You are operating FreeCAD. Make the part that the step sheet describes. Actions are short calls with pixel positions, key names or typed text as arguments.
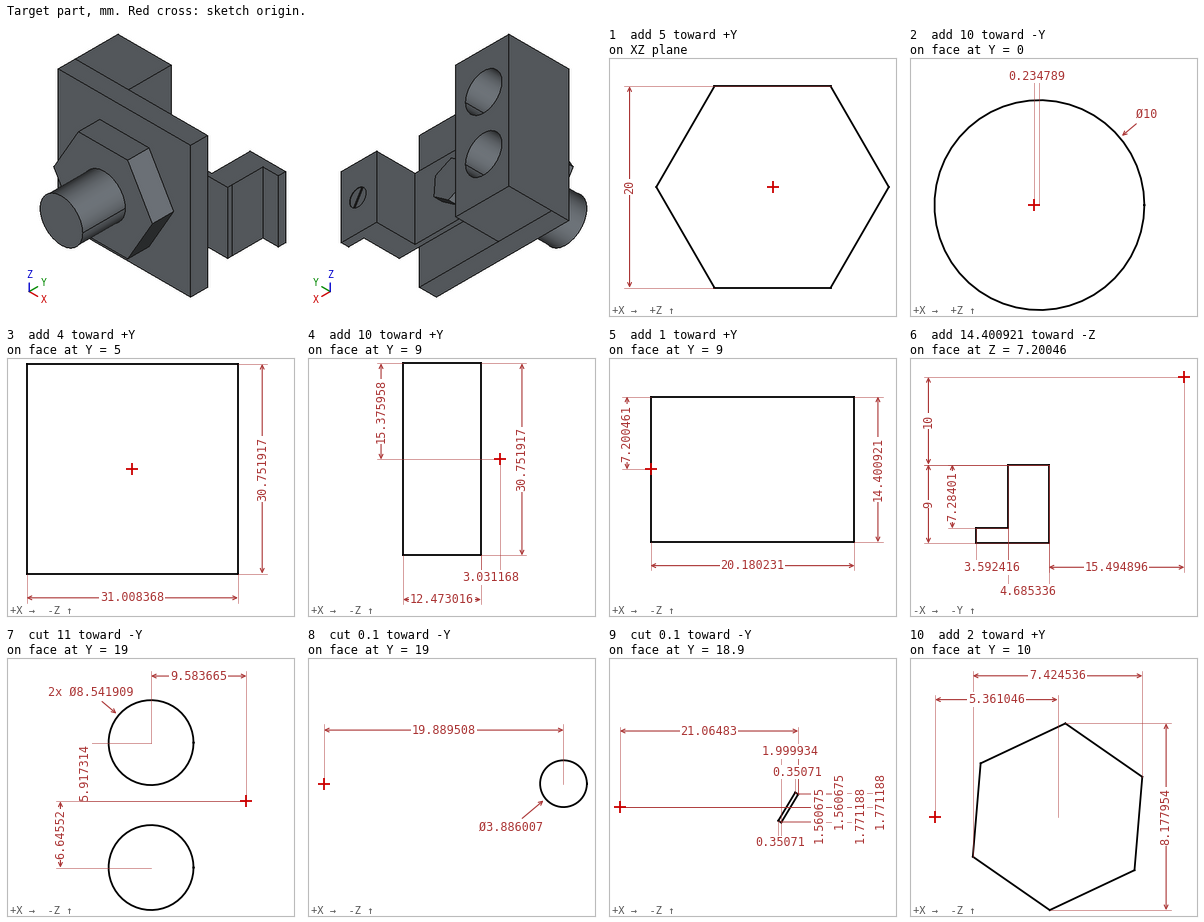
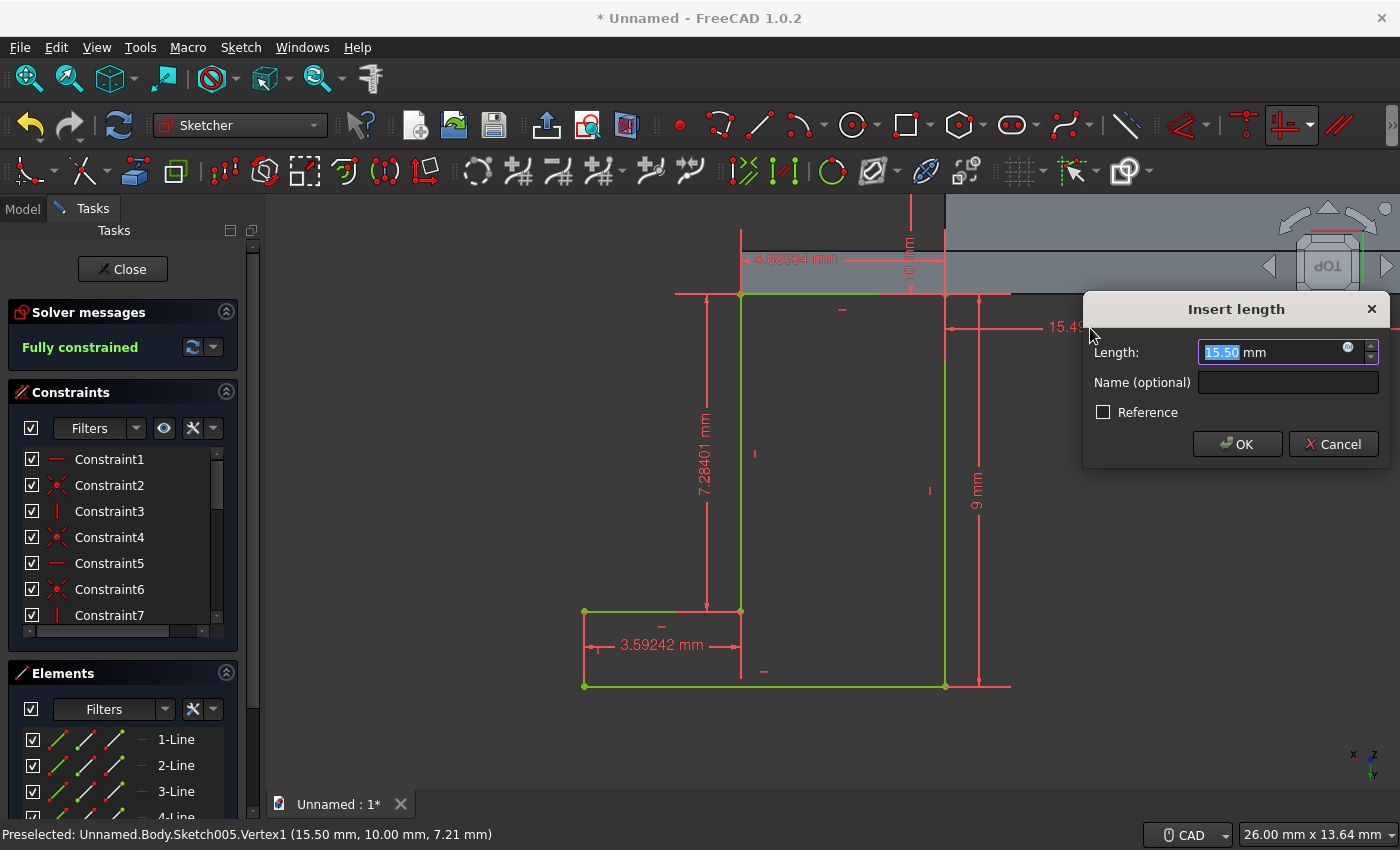
text(15.494896)
key(Return)
key(Escape)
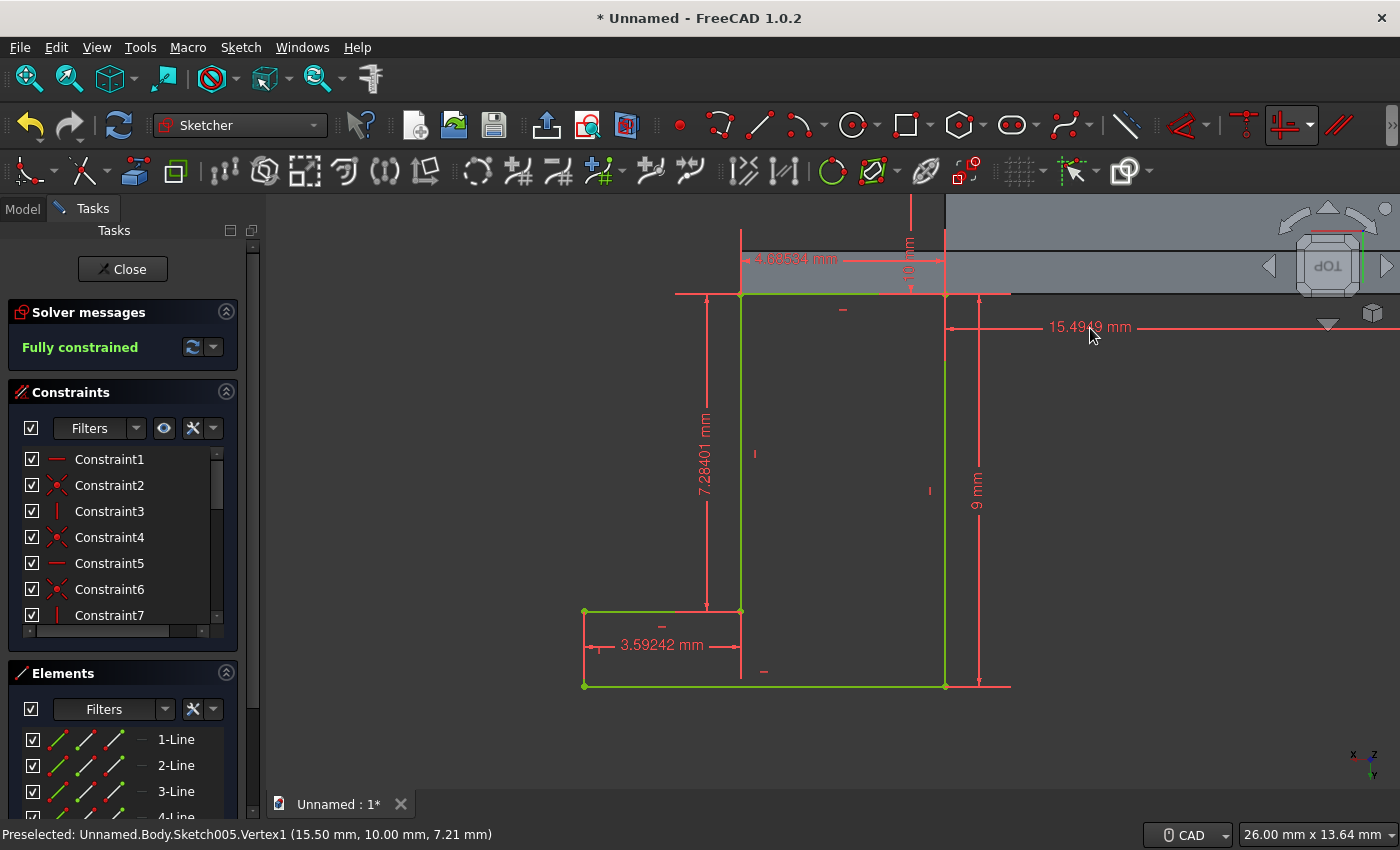
click(123, 269)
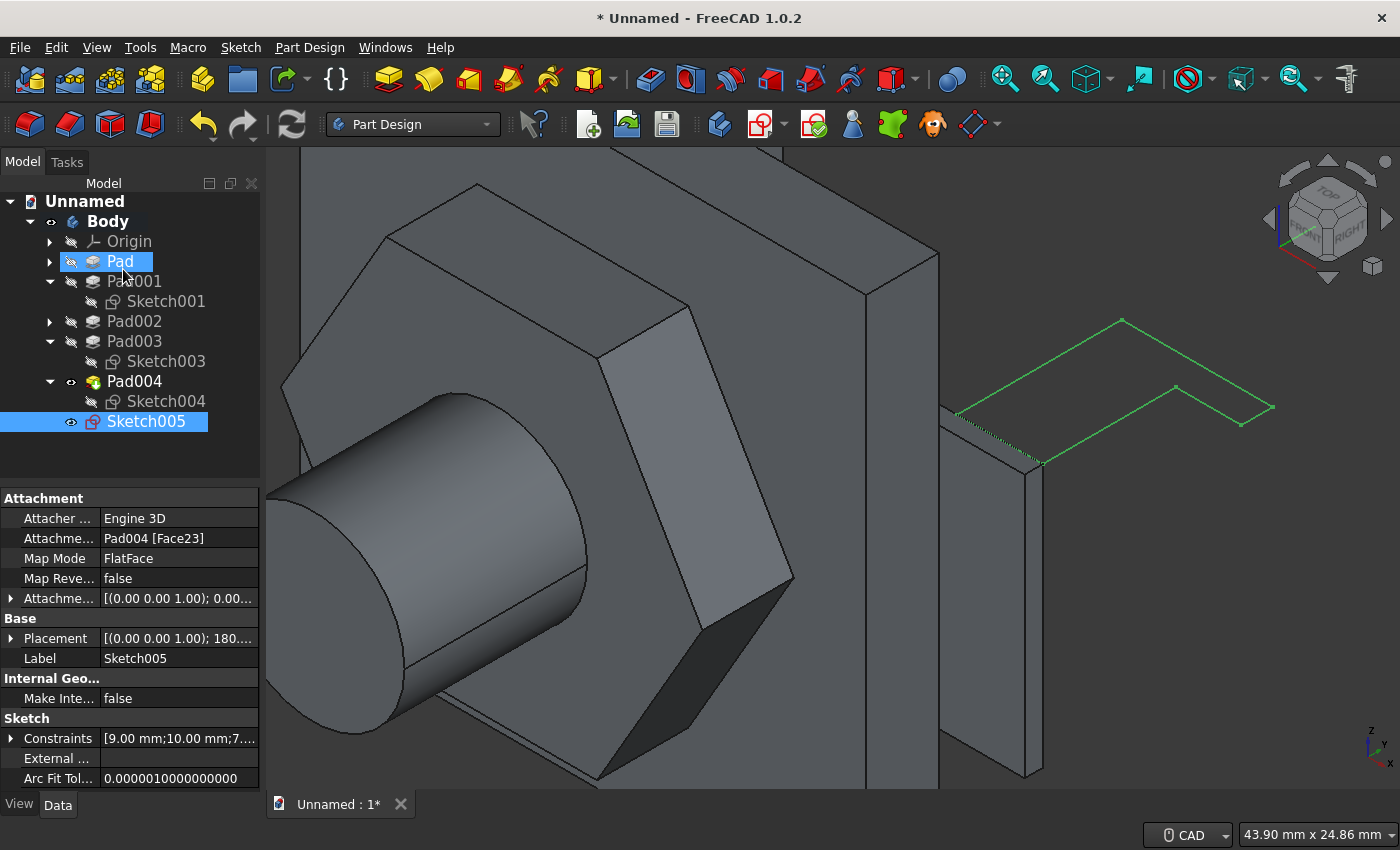
click(390, 80)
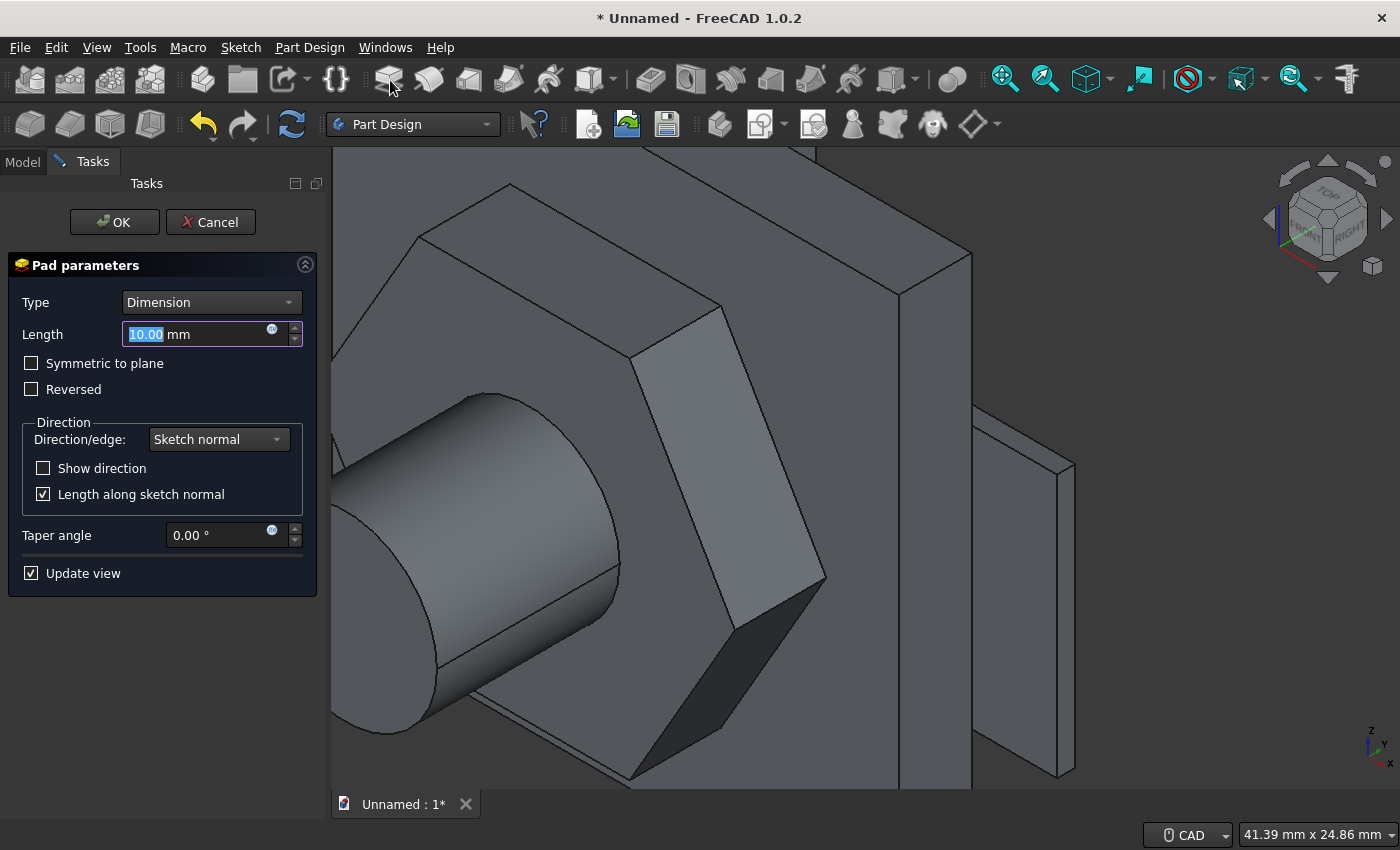
text(14.400921)
key(Tab)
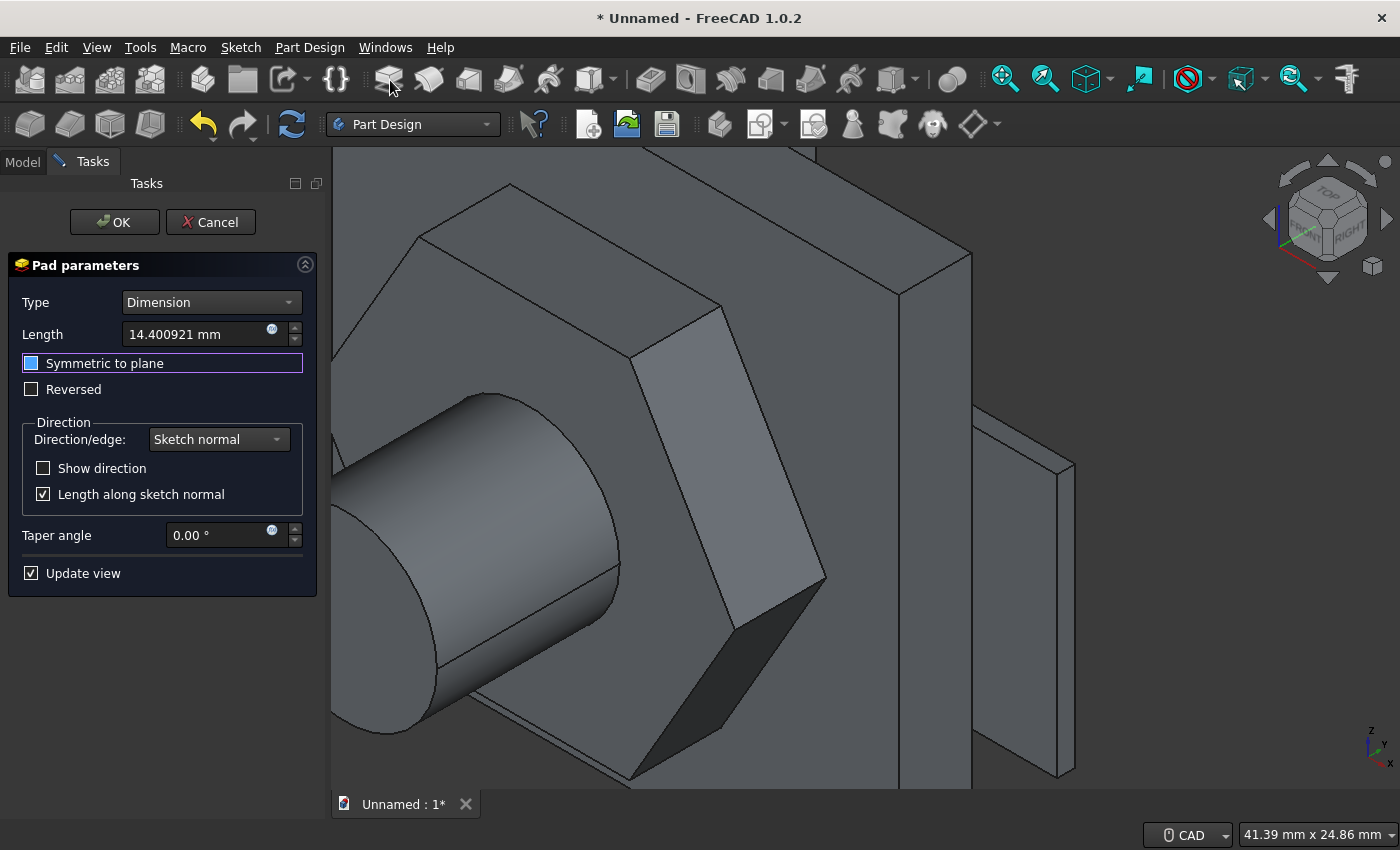
click(30, 389)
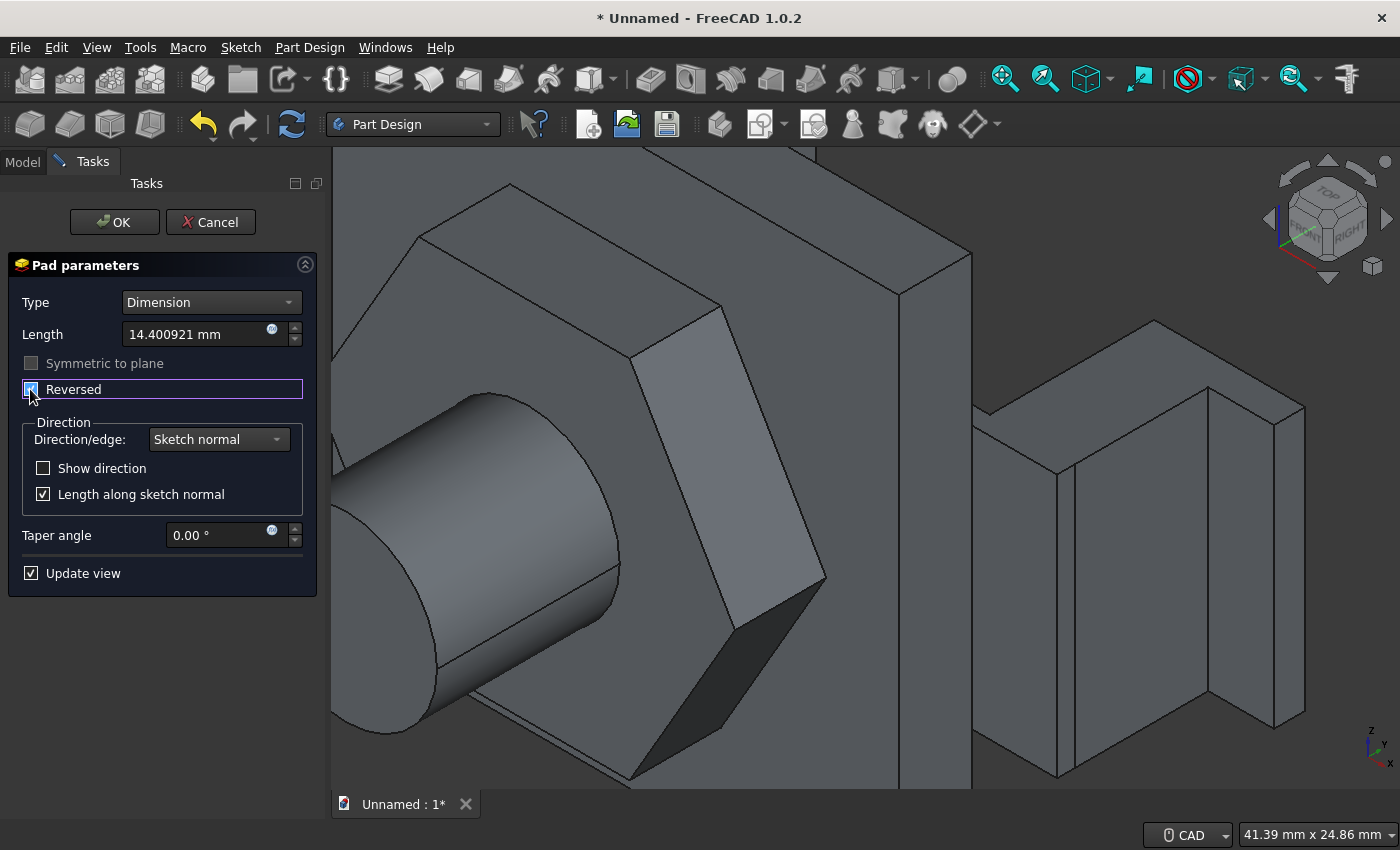
click(115, 222)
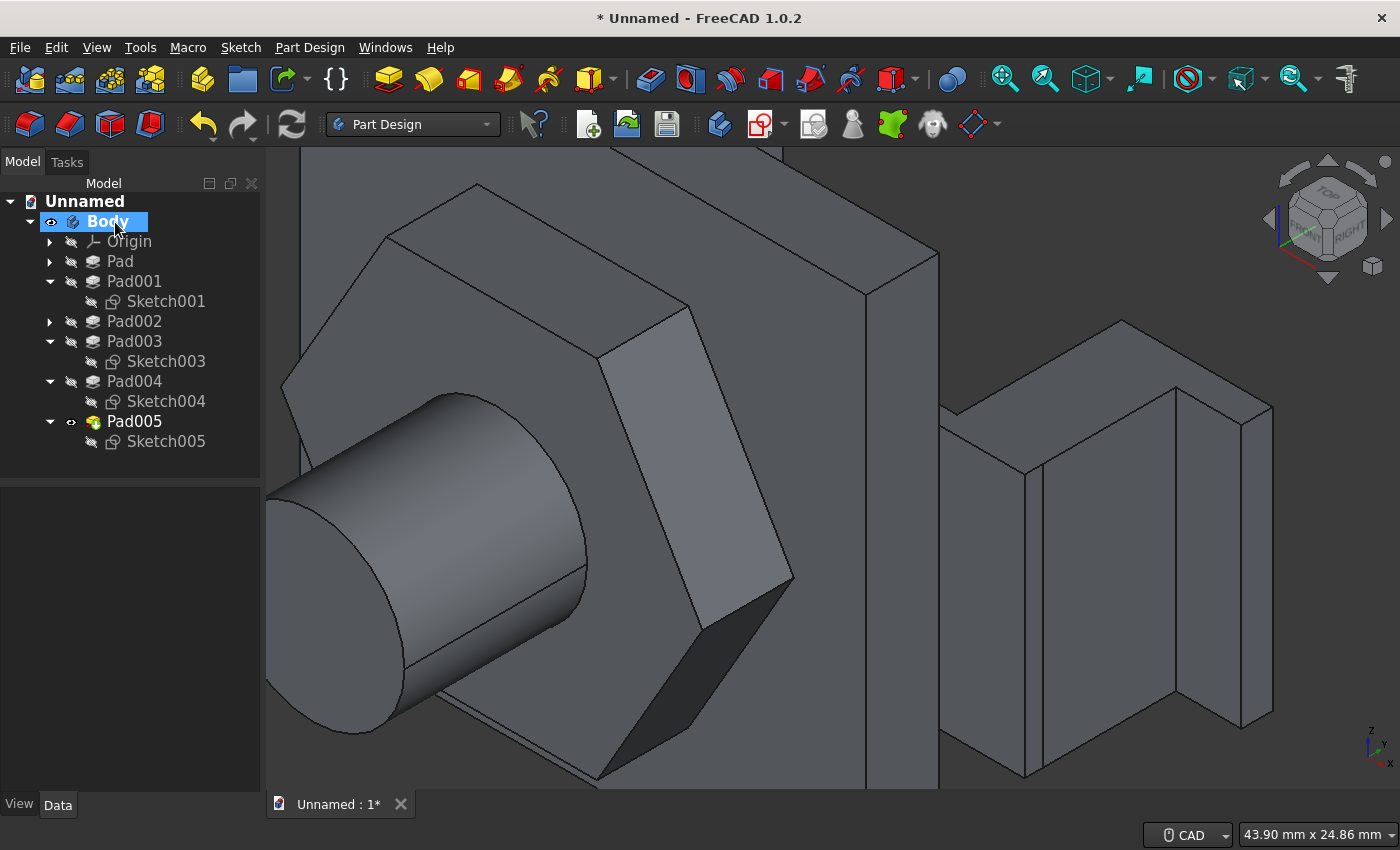
click(1006, 80)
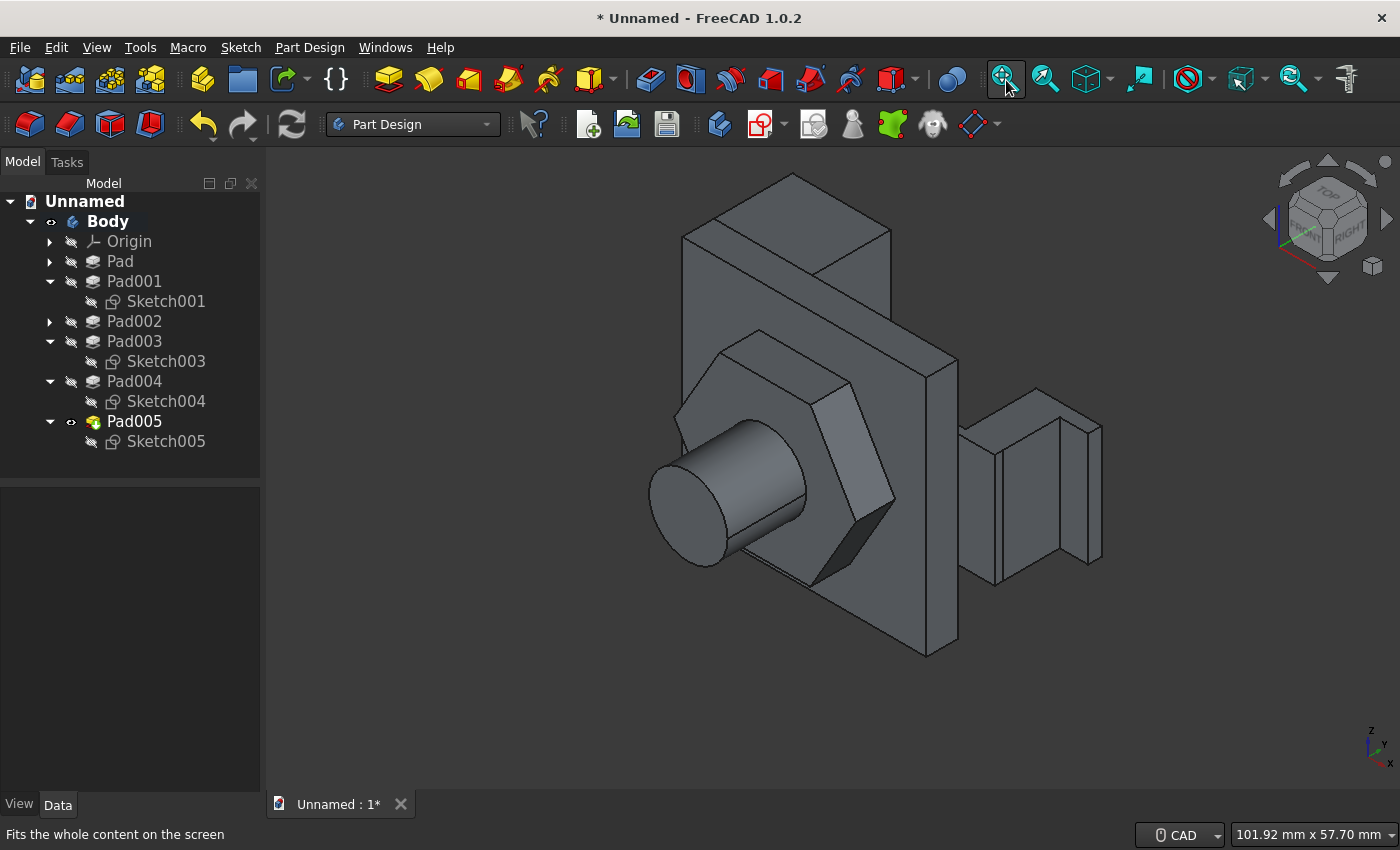
key(4)